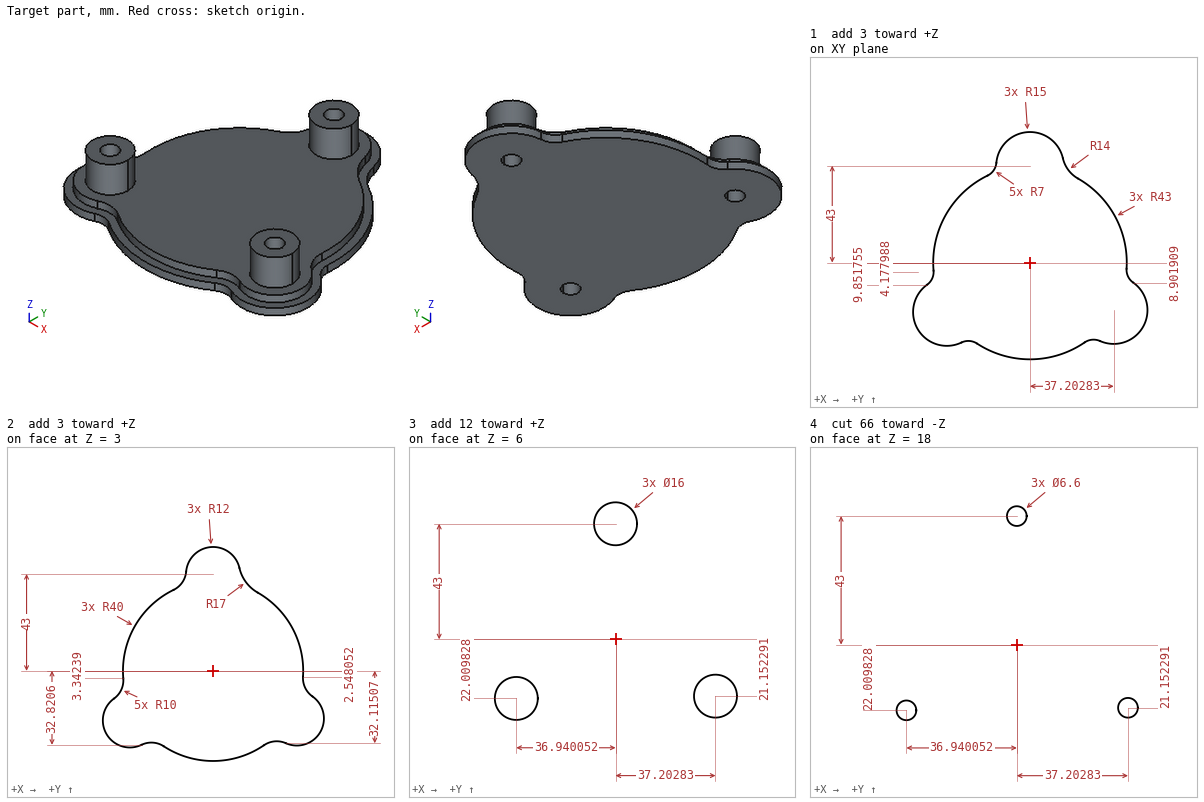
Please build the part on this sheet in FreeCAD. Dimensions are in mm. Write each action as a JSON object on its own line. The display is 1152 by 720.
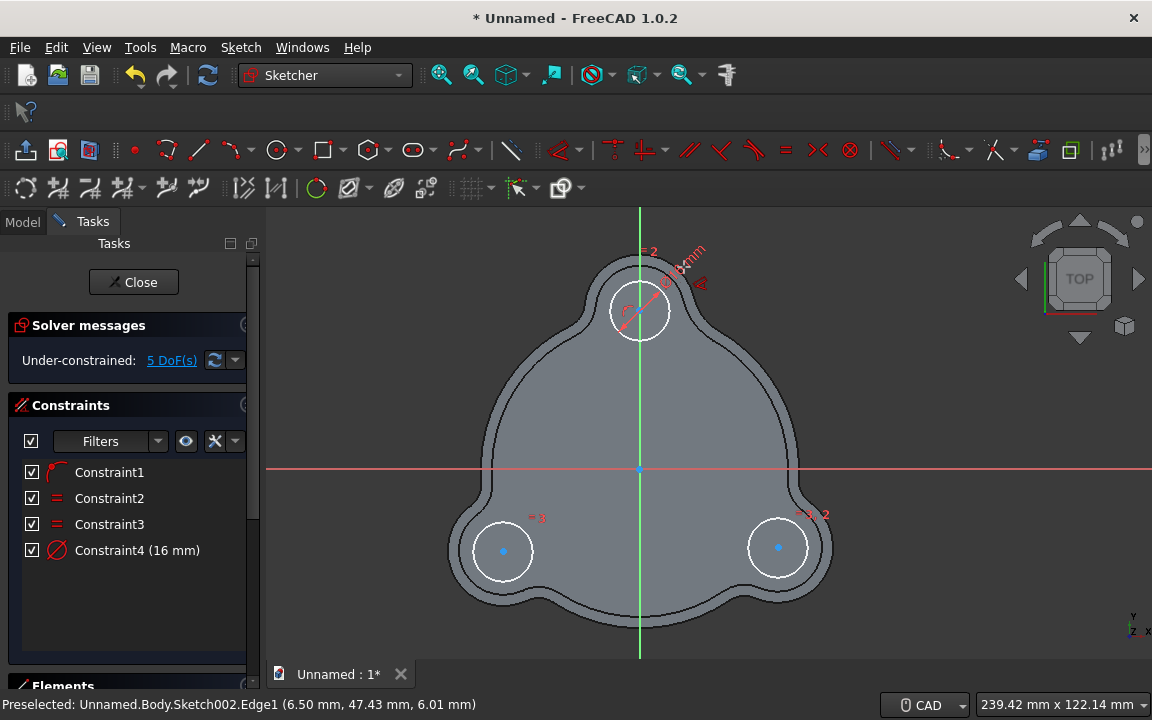
{"action": "left_click", "coordinate": [640, 311]}
{"action": "left_click", "coordinate": [606, 390]}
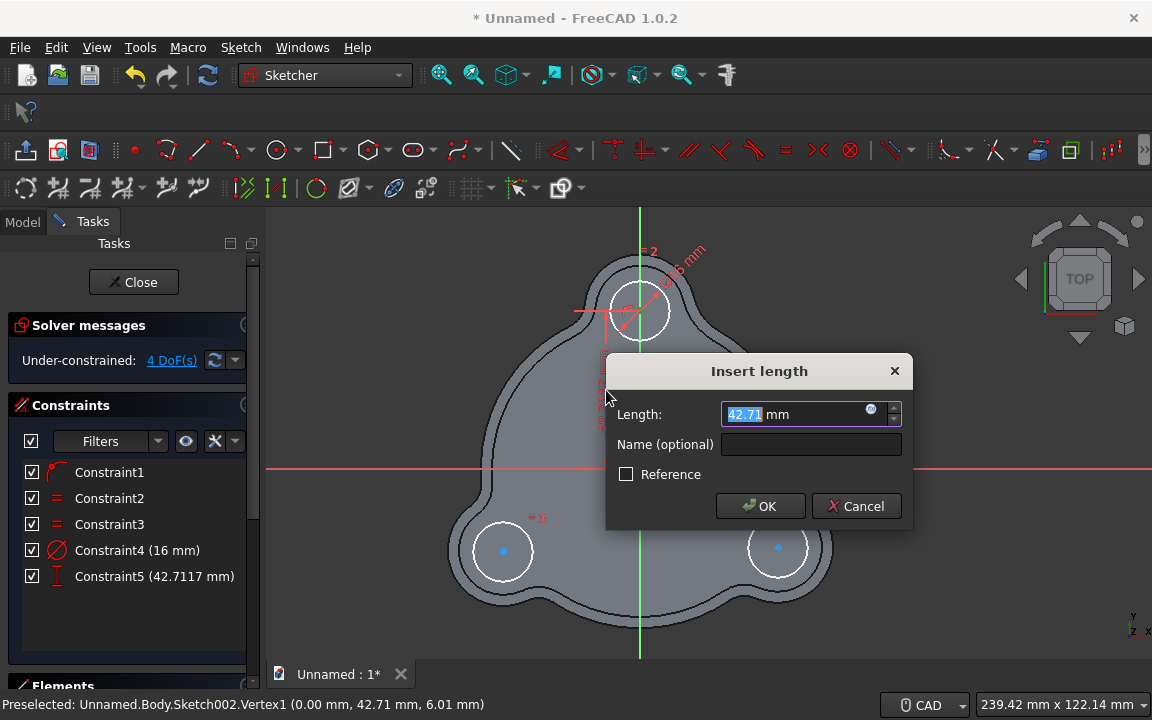
{"action": "type", "text": "43"}
{"action": "key", "text": "Return"}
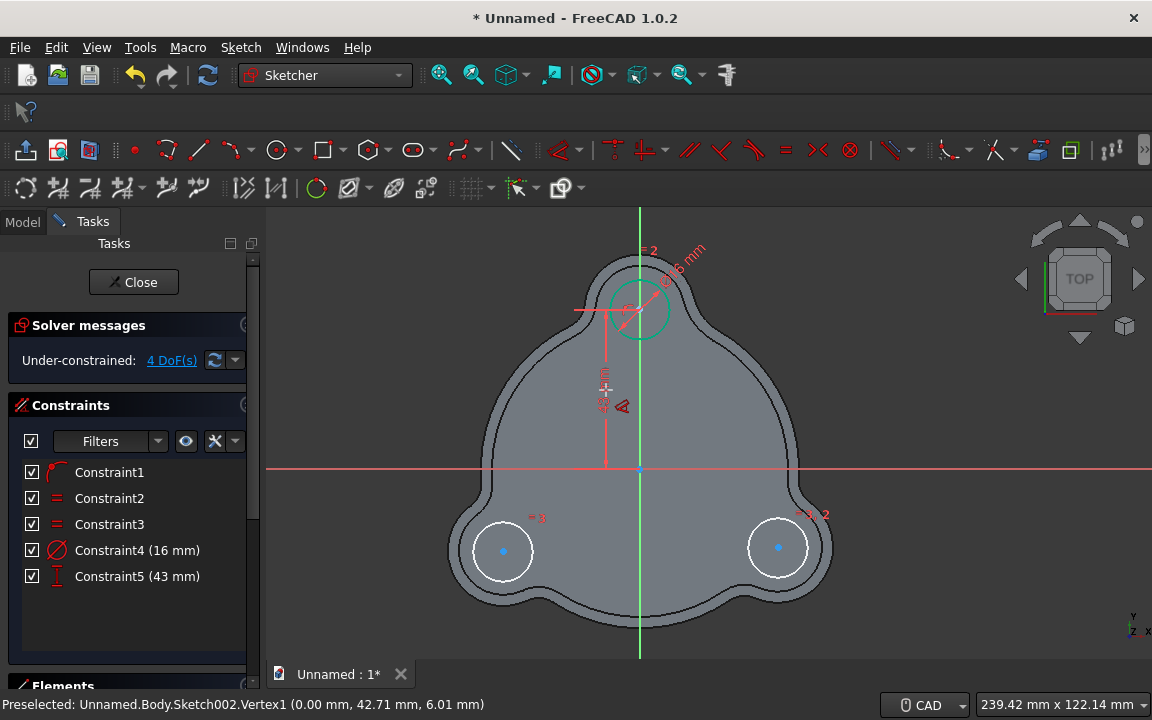
{"action": "left_click", "coordinate": [778, 548]}
{"action": "left_click", "coordinate": [709, 582]}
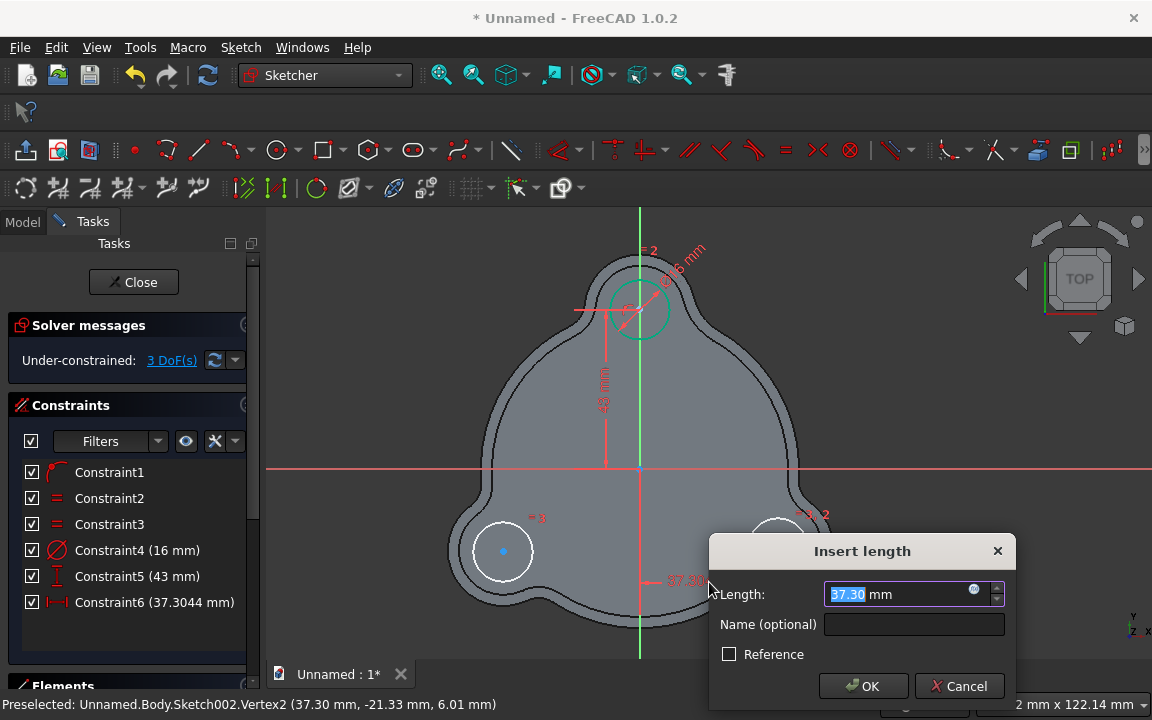
{"action": "type", "text": "37.20283"}
{"action": "key", "text": "Return"}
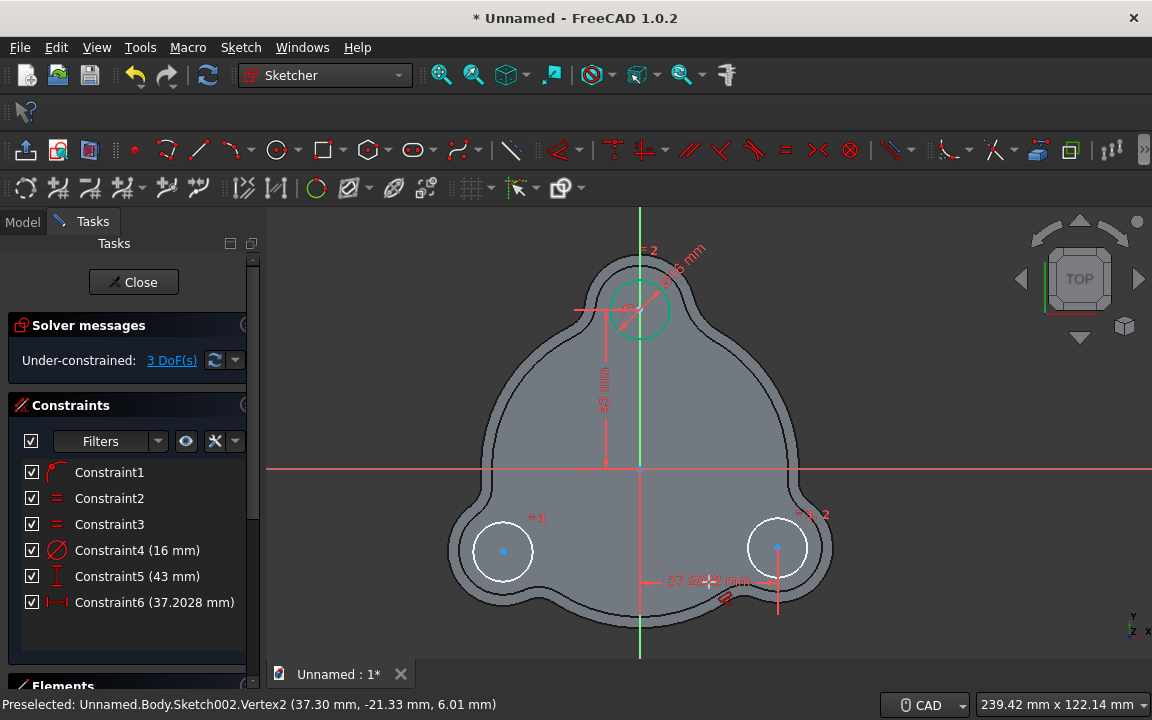
{"action": "left_click", "coordinate": [778, 548]}
{"action": "left_click", "coordinate": [812, 509]}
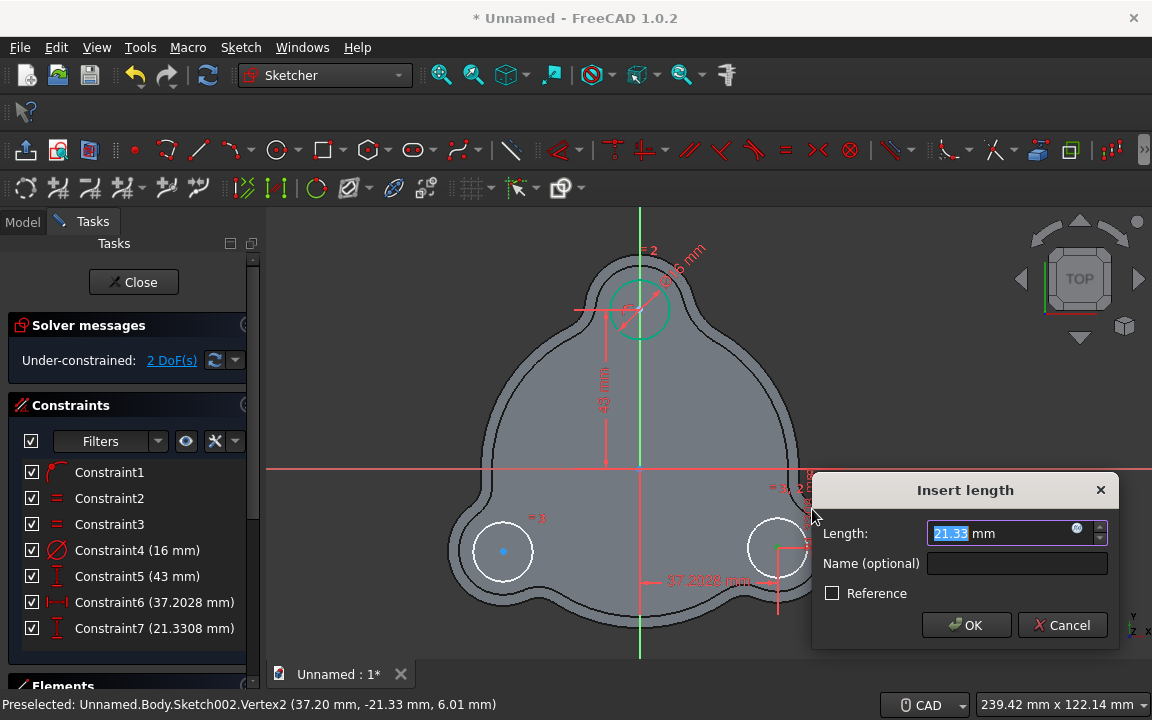
{"action": "type", "text": "21.152291"}
{"action": "key", "text": "Return"}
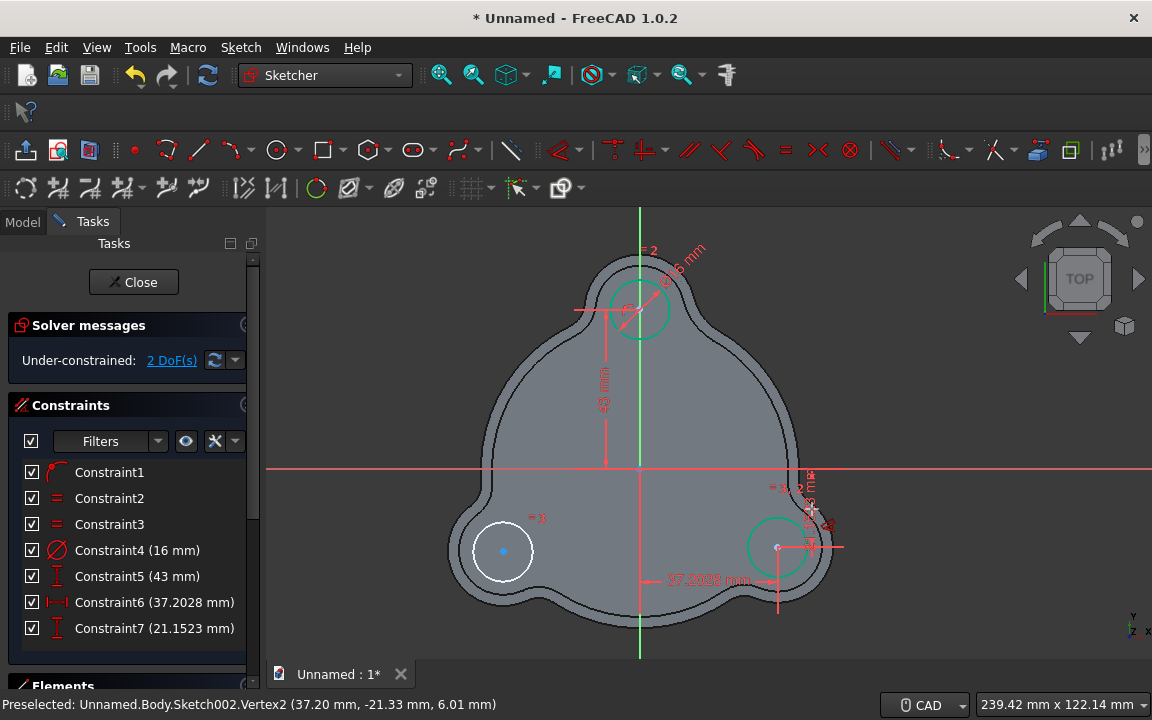
{"action": "left_click", "coordinate": [503, 552]}
{"action": "left_click", "coordinate": [571, 586]}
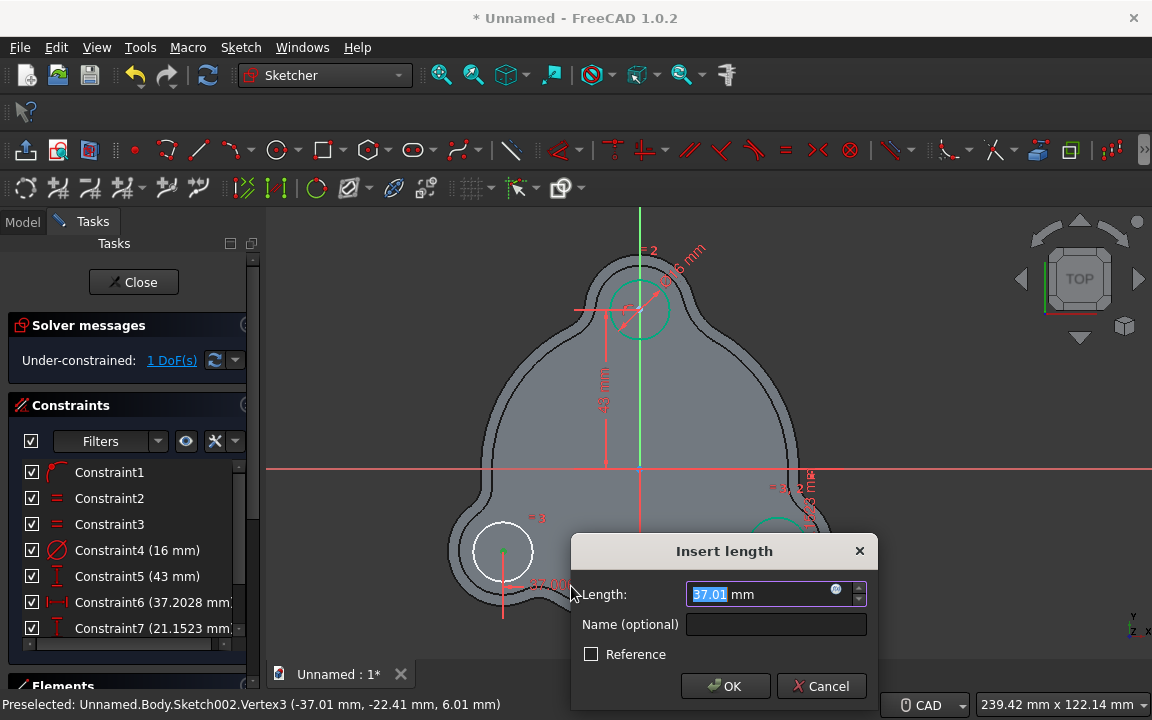
{"action": "type", "text": "36.940052"}
{"action": "key", "text": "Return"}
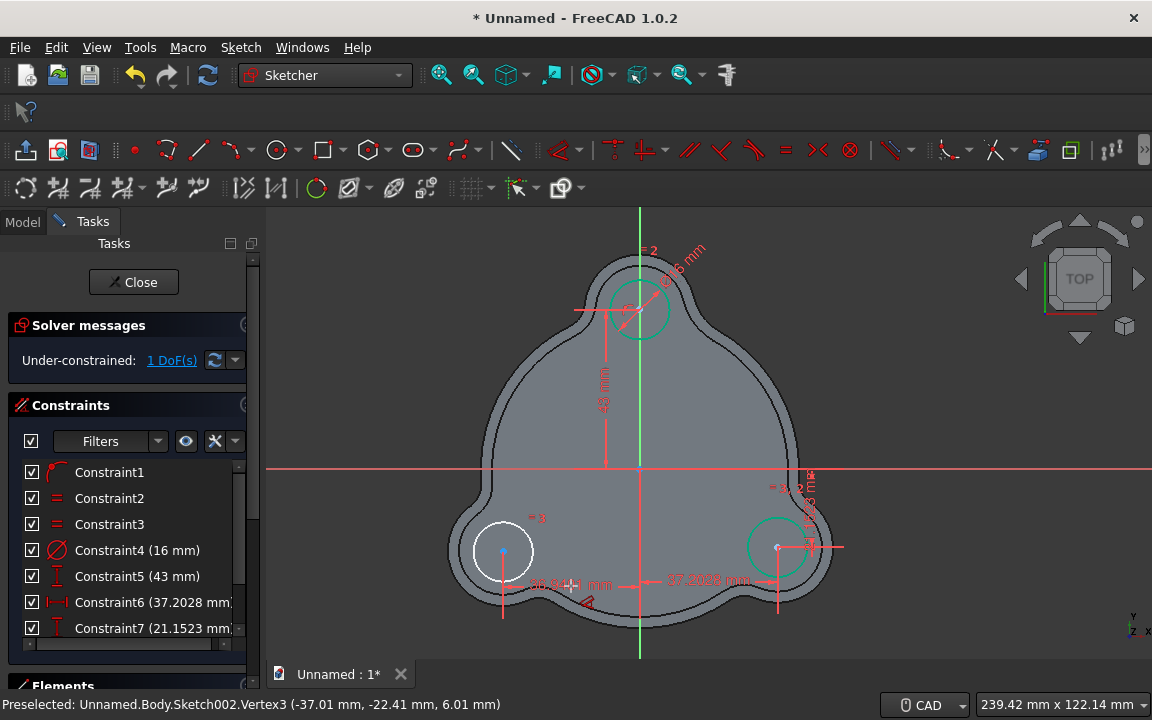
{"action": "left_click", "coordinate": [503, 552]}
{"action": "left_click", "coordinate": [469, 511]}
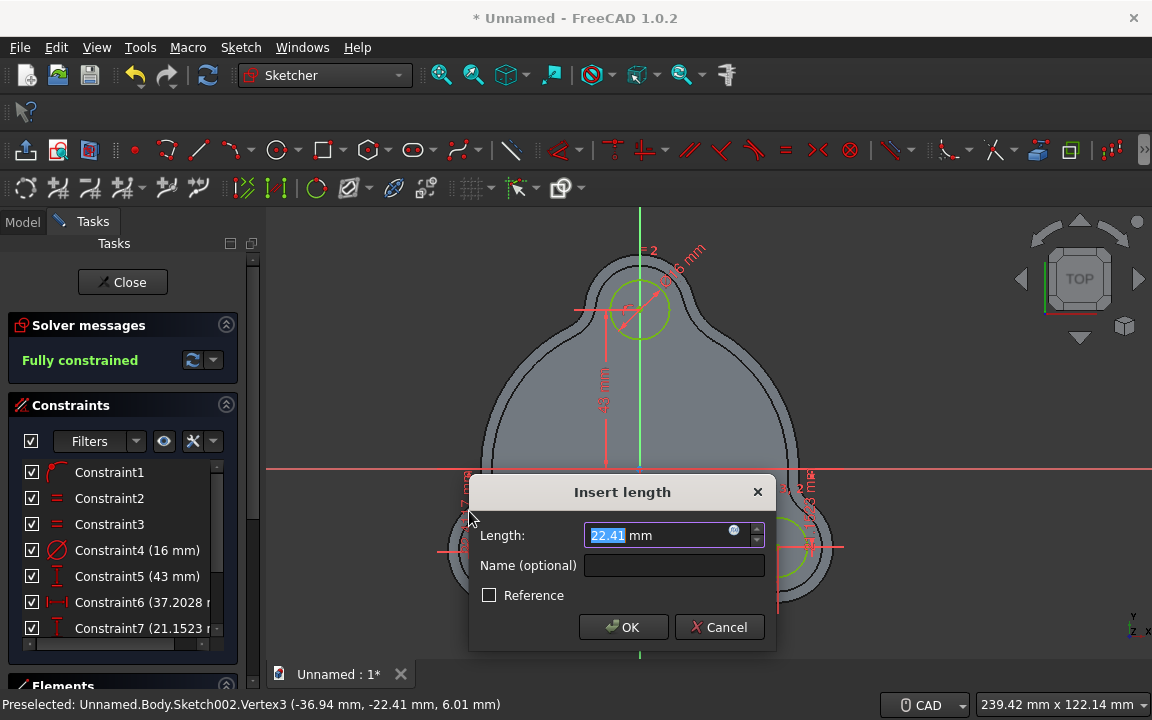
{"action": "type", "text": "22.009828"}
{"action": "key", "text": "Return"}
{"action": "key", "text": "Escape"}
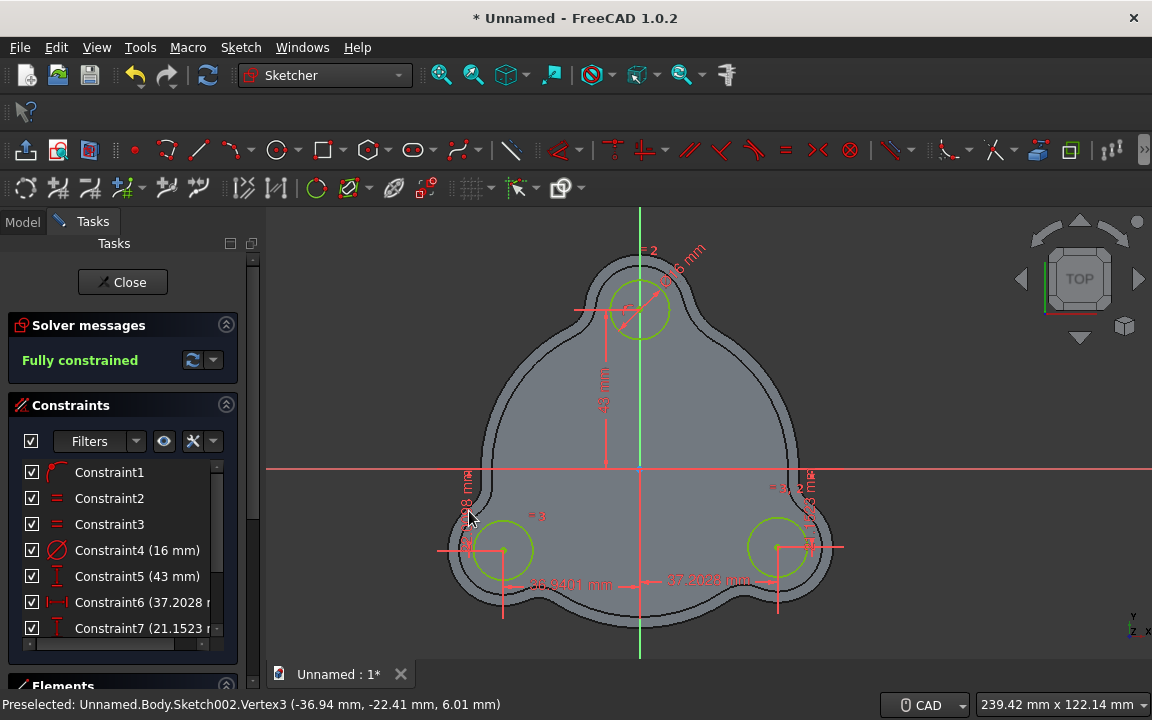
{"action": "left_click", "coordinate": [123, 282]}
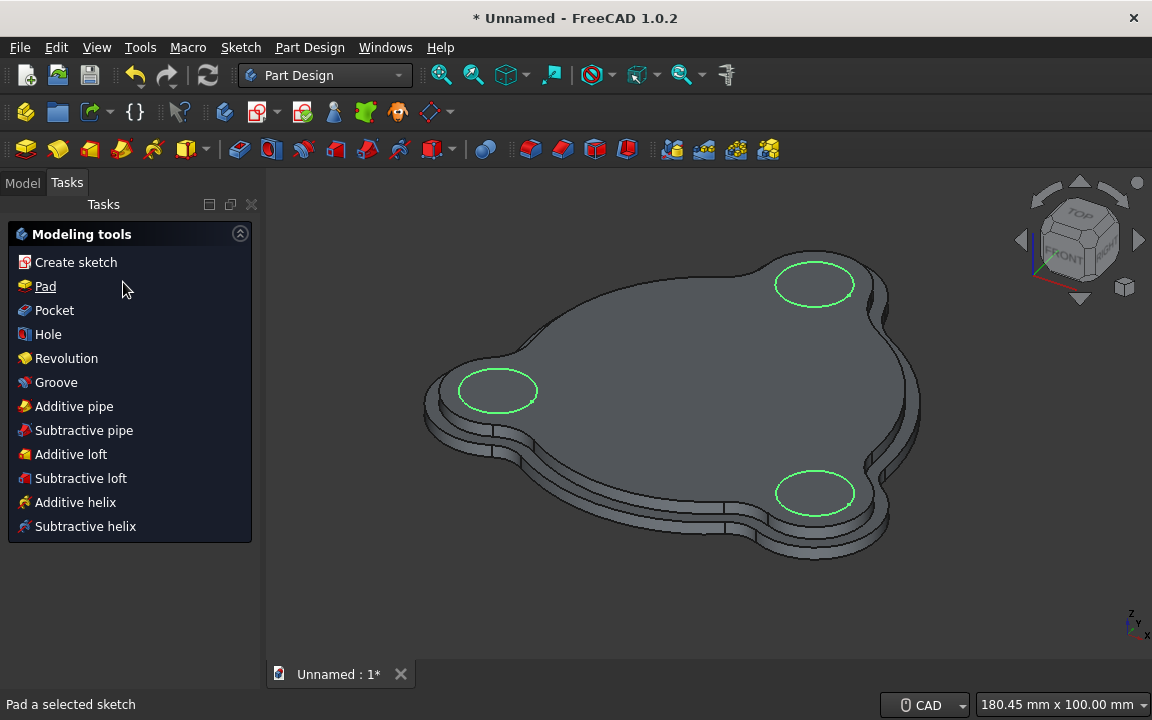
{"action": "left_click", "coordinate": [26, 150]}